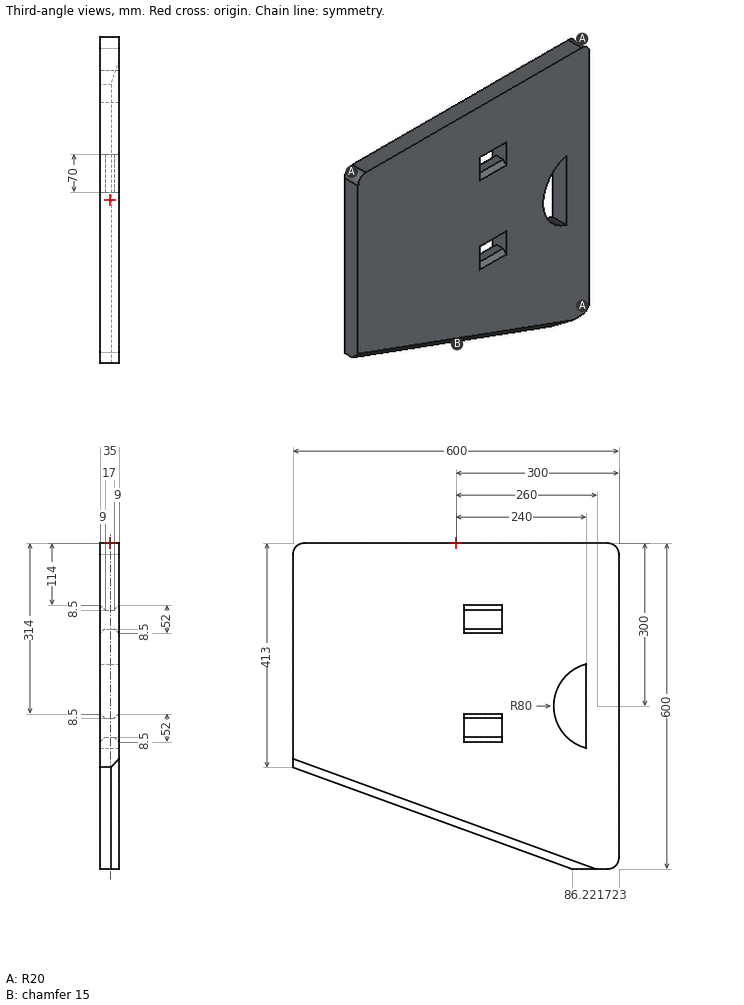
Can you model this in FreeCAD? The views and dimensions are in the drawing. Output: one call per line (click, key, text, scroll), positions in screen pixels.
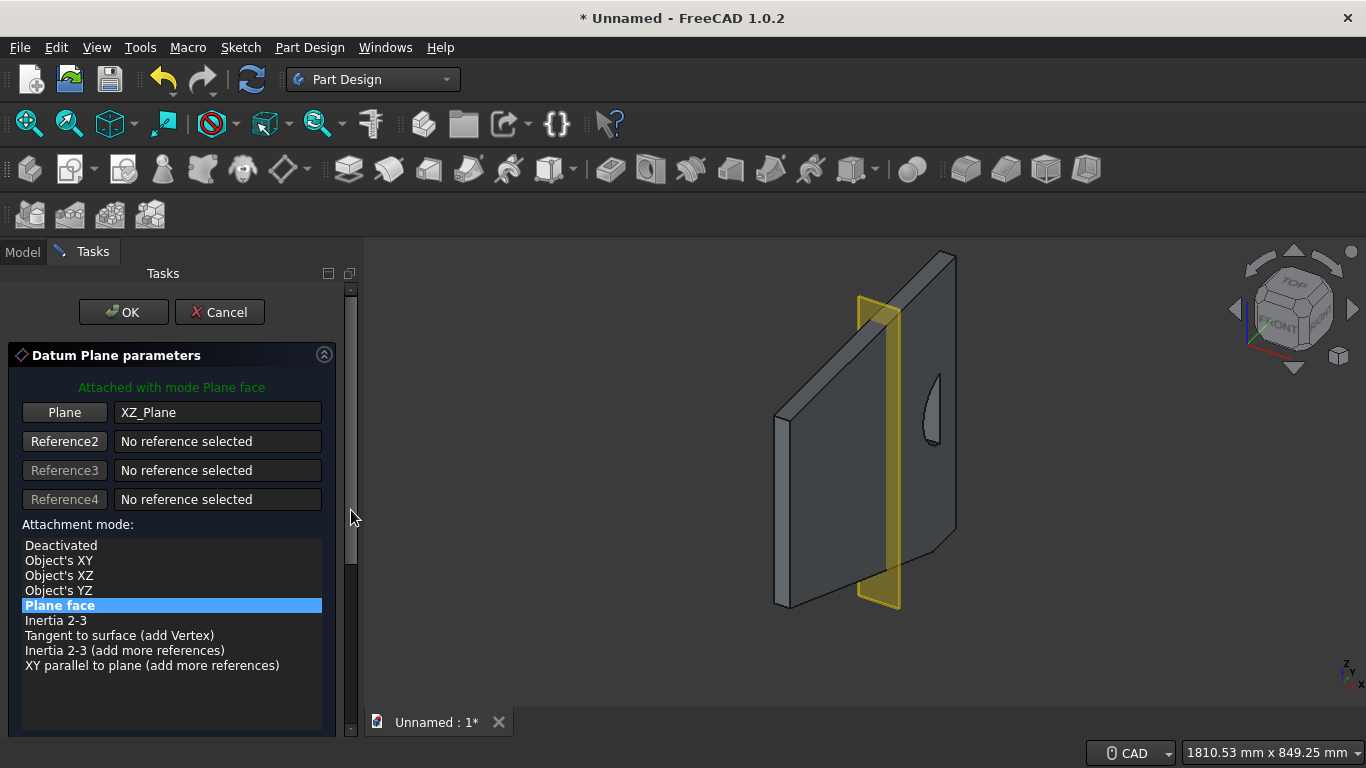
click(124, 312)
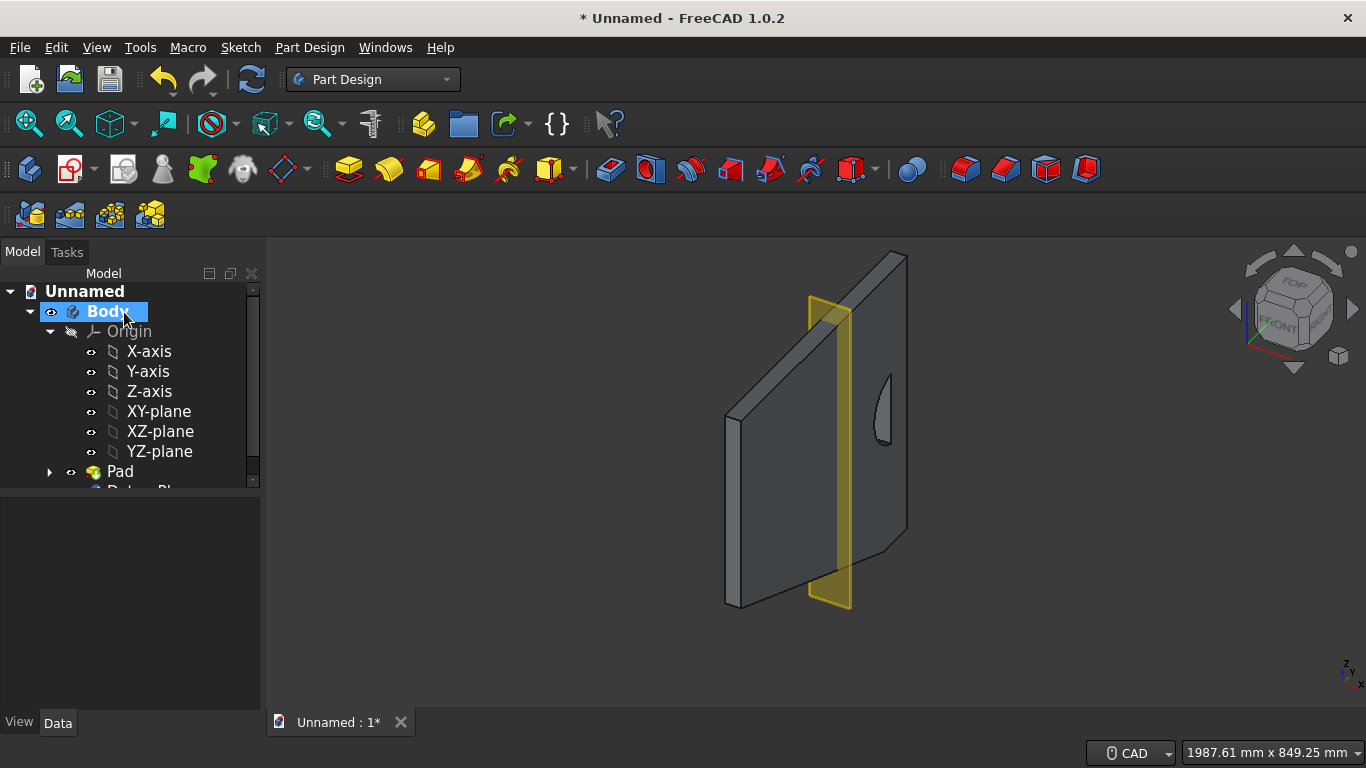
scroll(100, 387, down, 3)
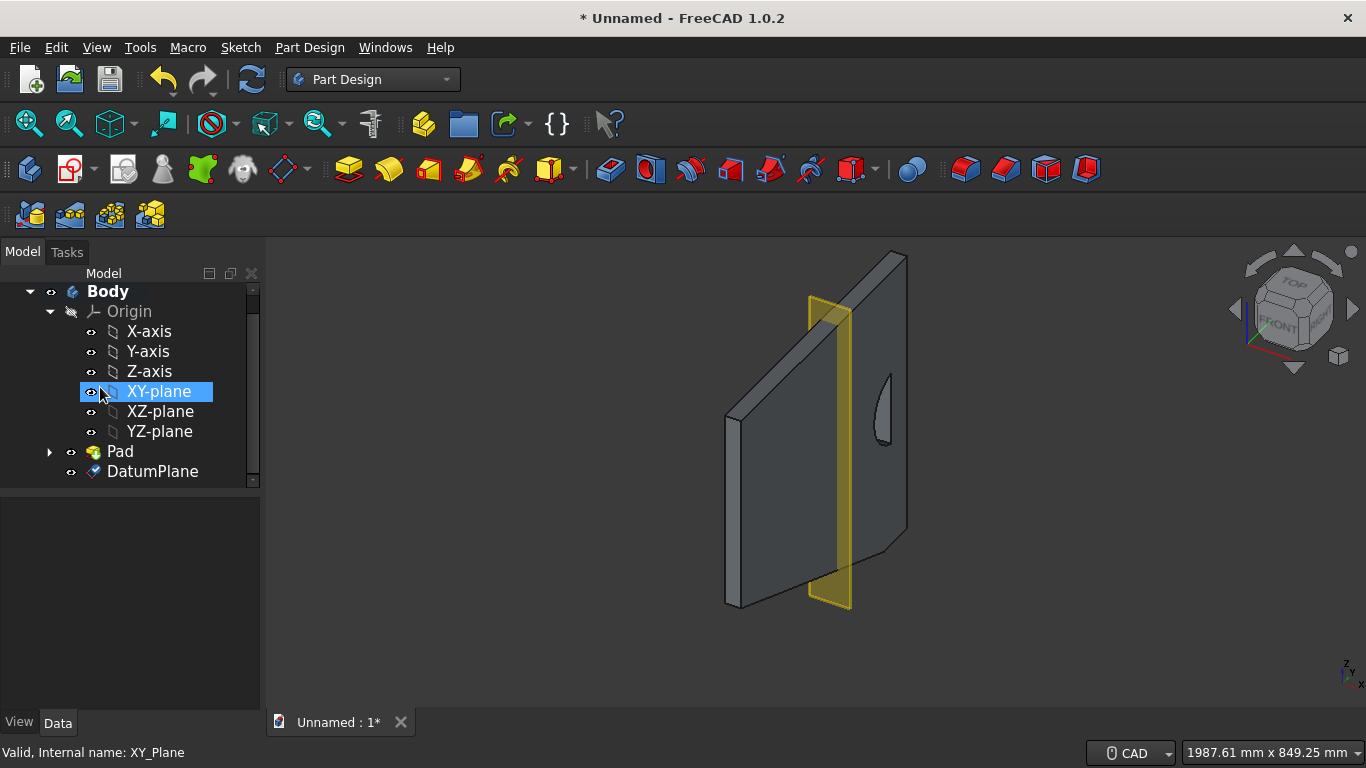
click(116, 472)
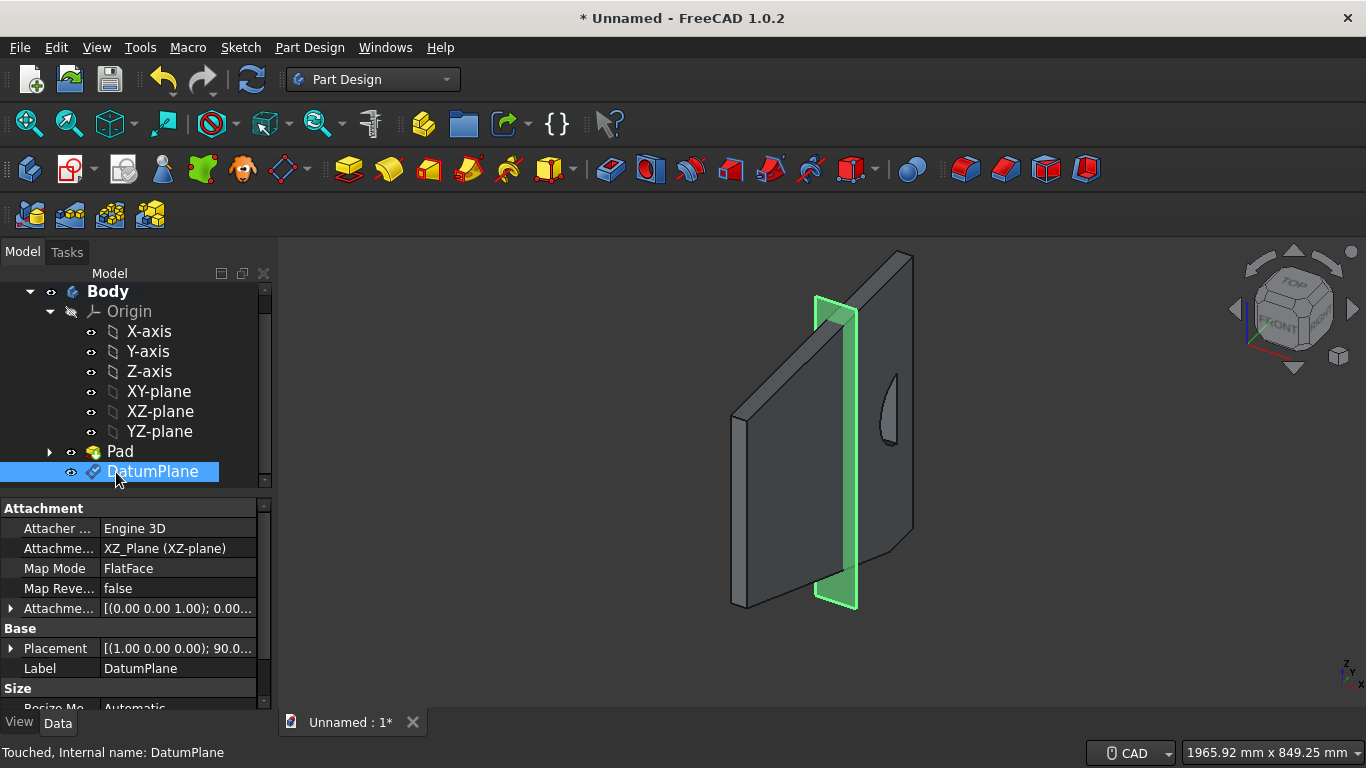
click(70, 170)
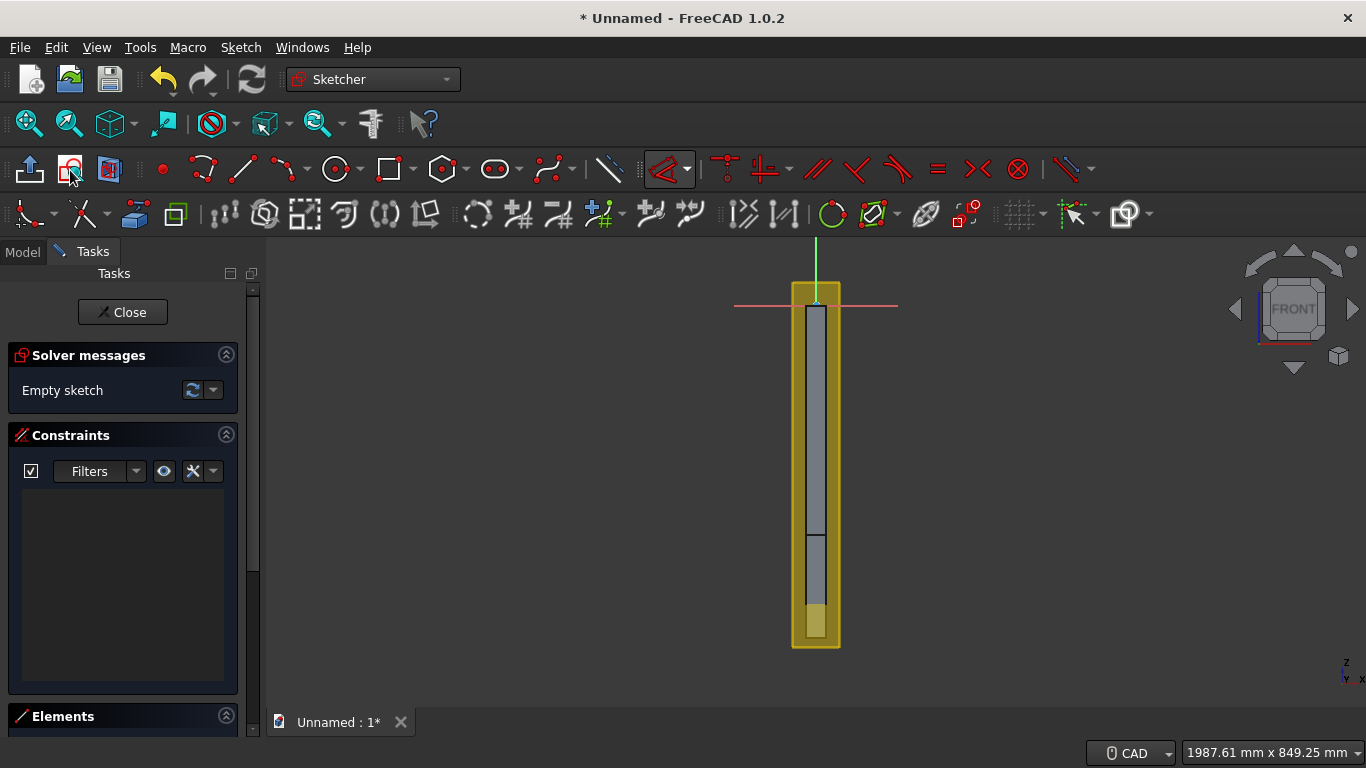
click(110, 170)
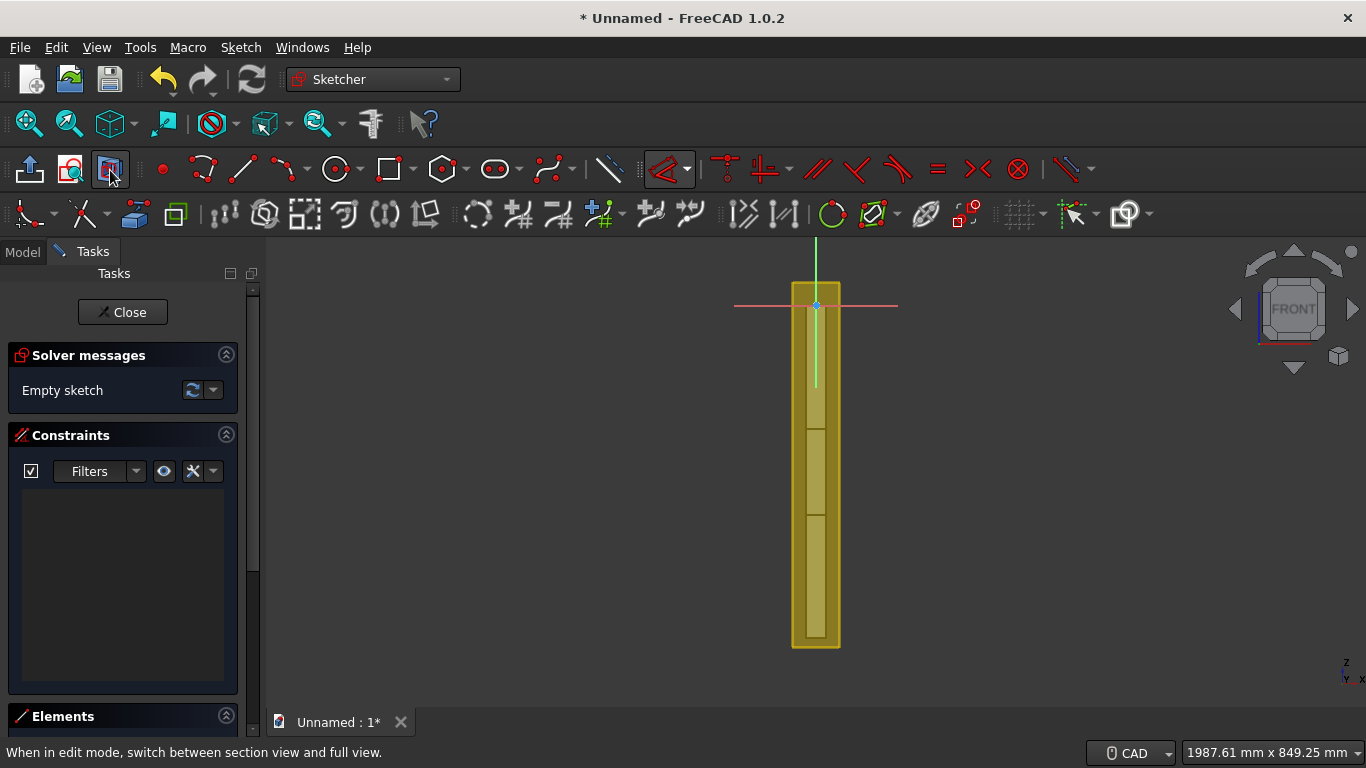
scroll(955, 276, up, 2)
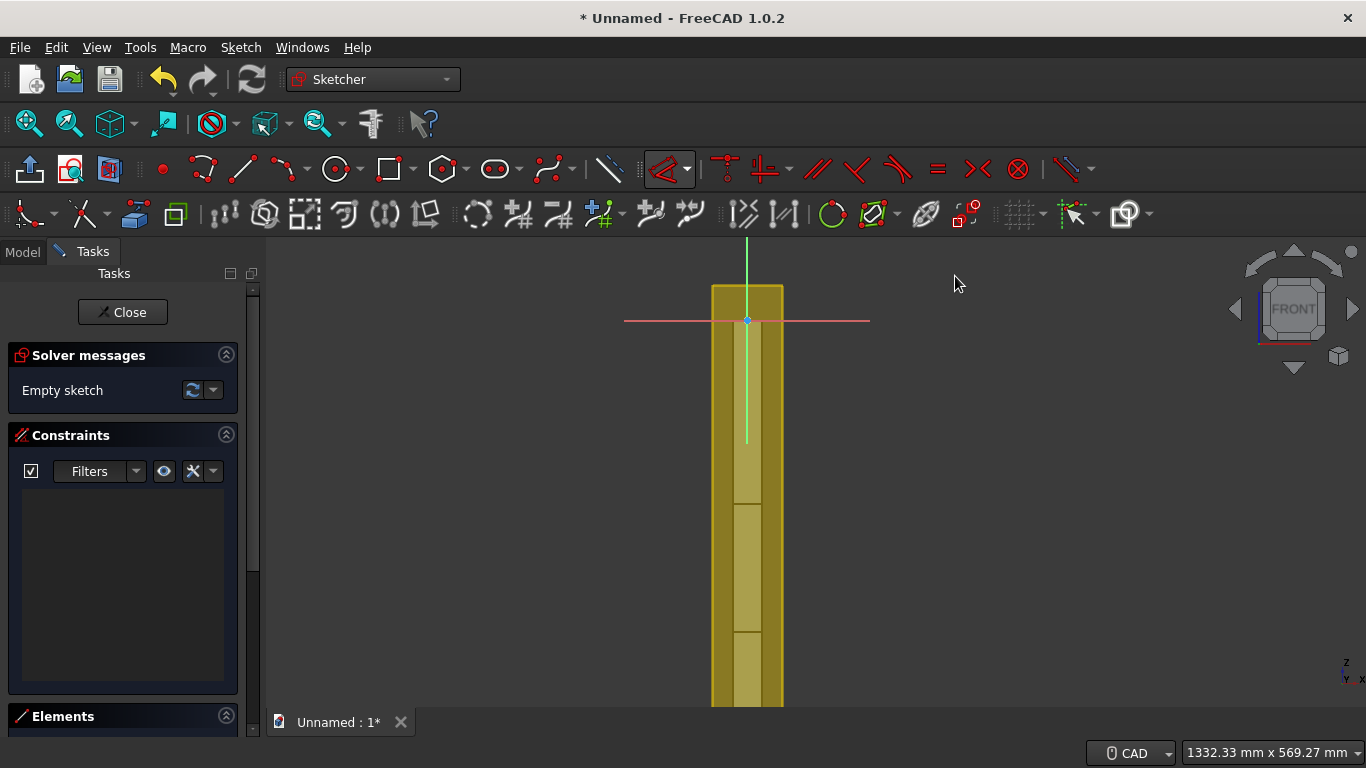
click(204, 170)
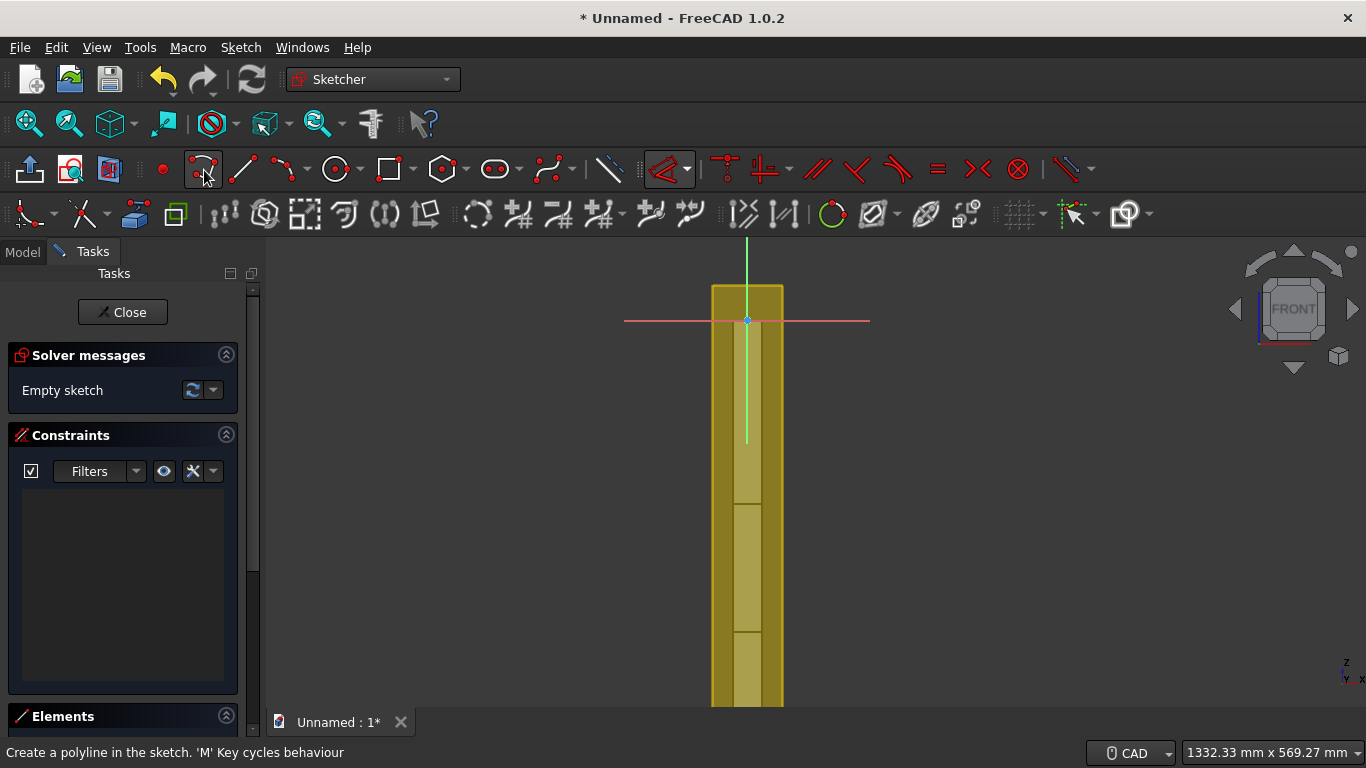
click(733, 415)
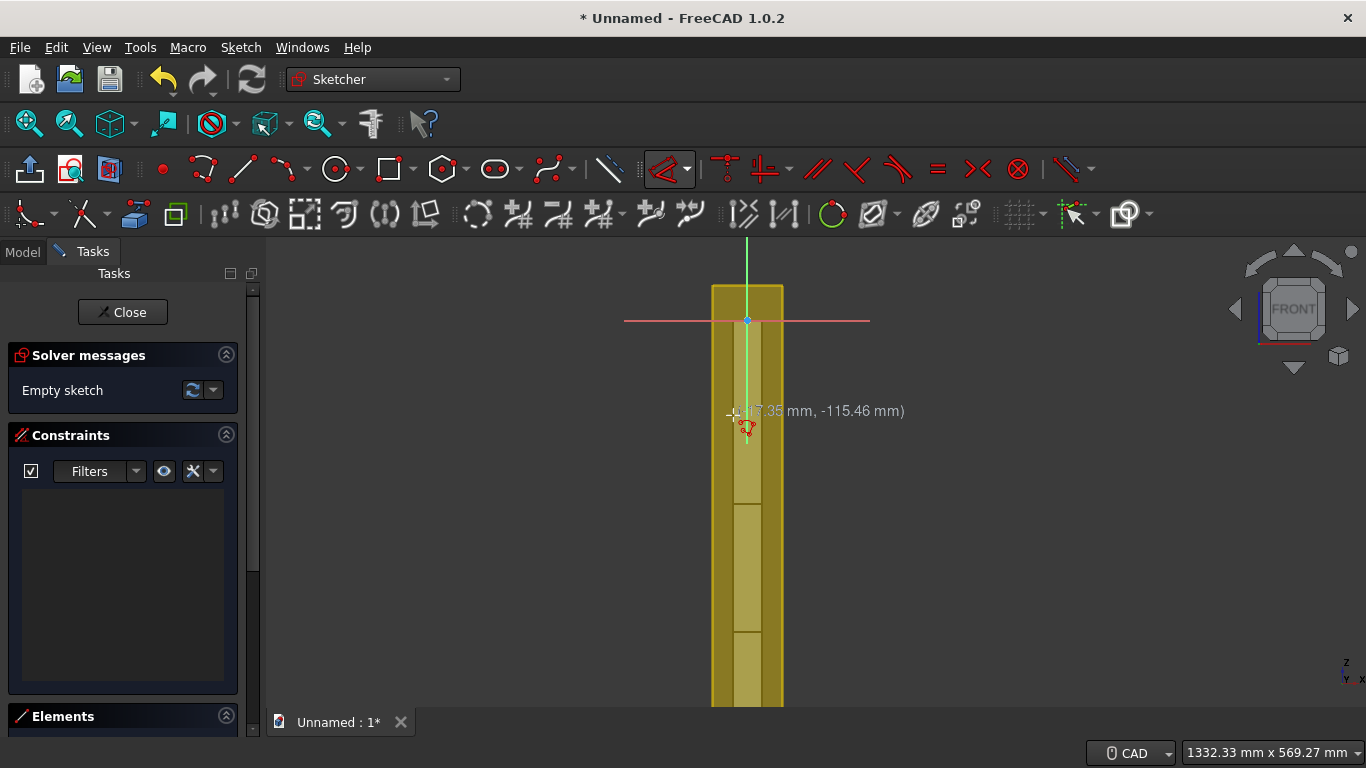
scroll(740, 422, up, 5)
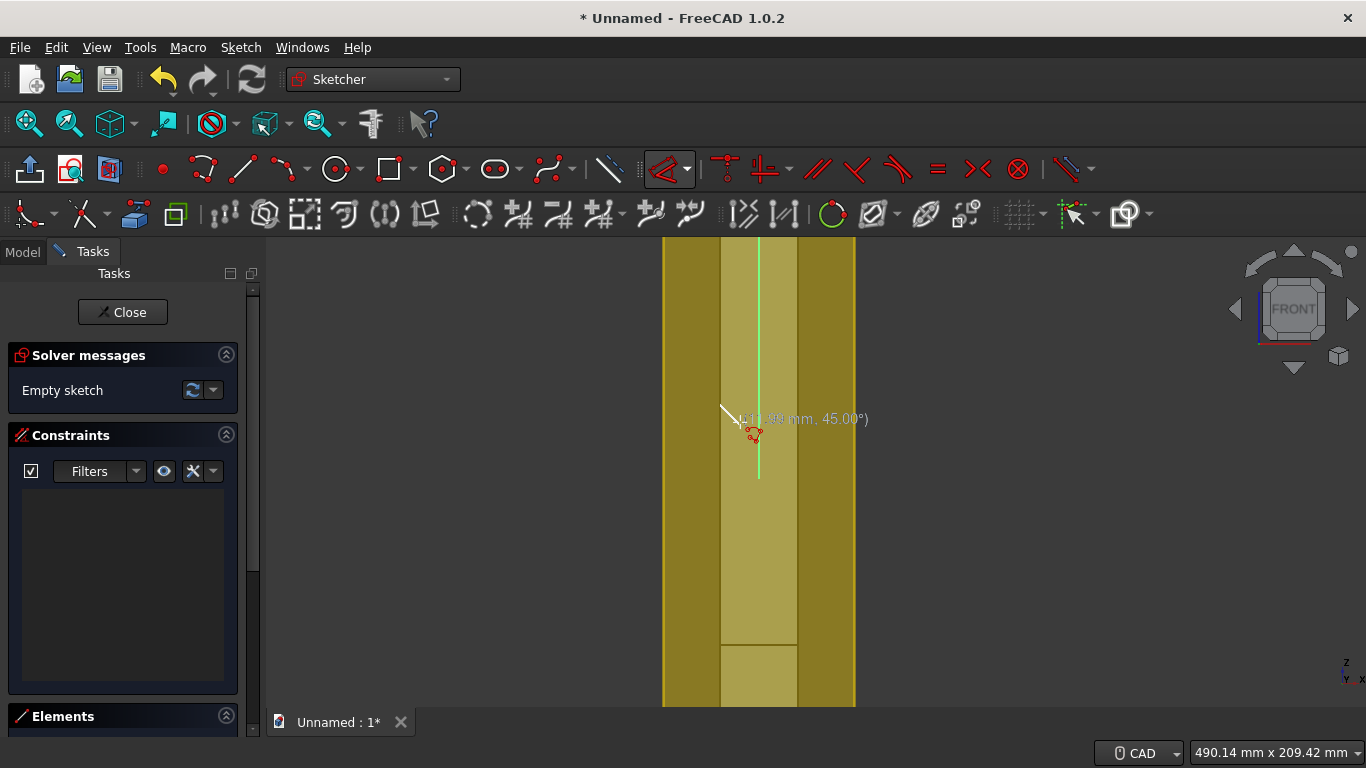
click(740, 421)
click(778, 421)
click(798, 402)
click(798, 518)
click(778, 499)
click(740, 499)
click(720, 518)
click(720, 405)